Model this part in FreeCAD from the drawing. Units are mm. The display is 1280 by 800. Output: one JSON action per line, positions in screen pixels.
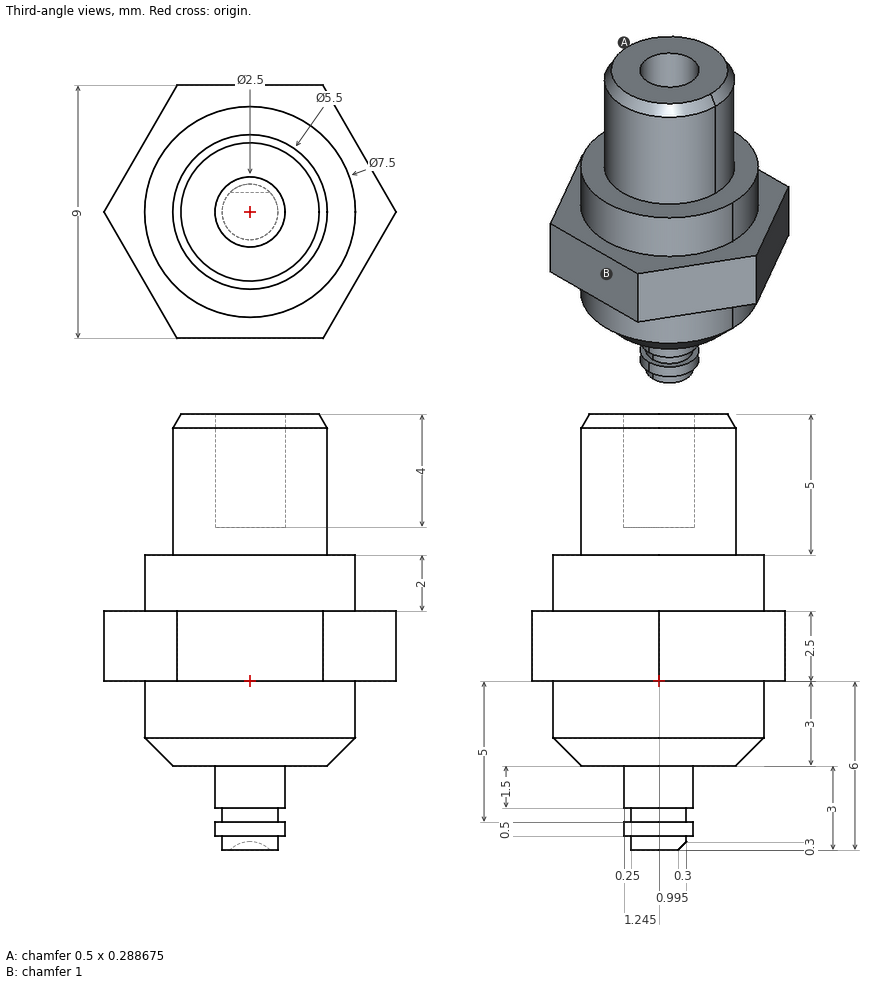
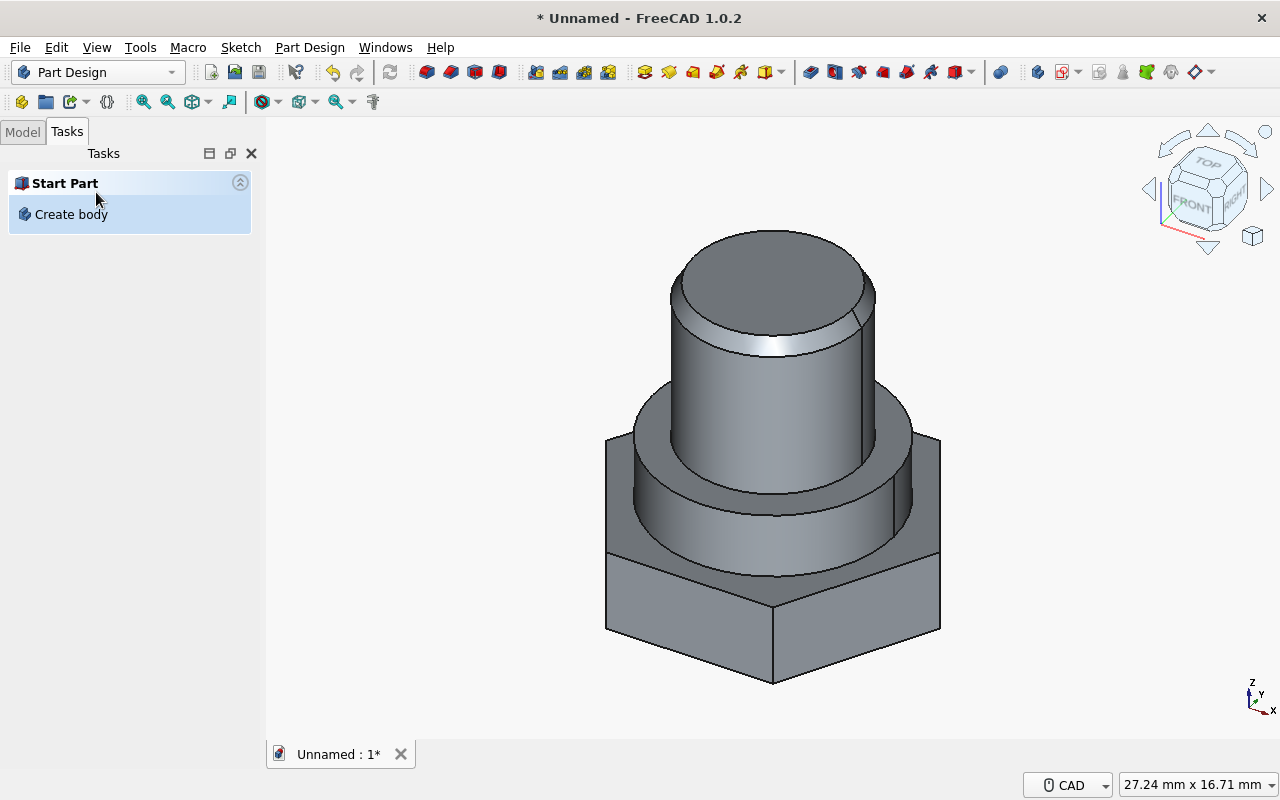
{"action": "left_click", "coordinate": [773, 282]}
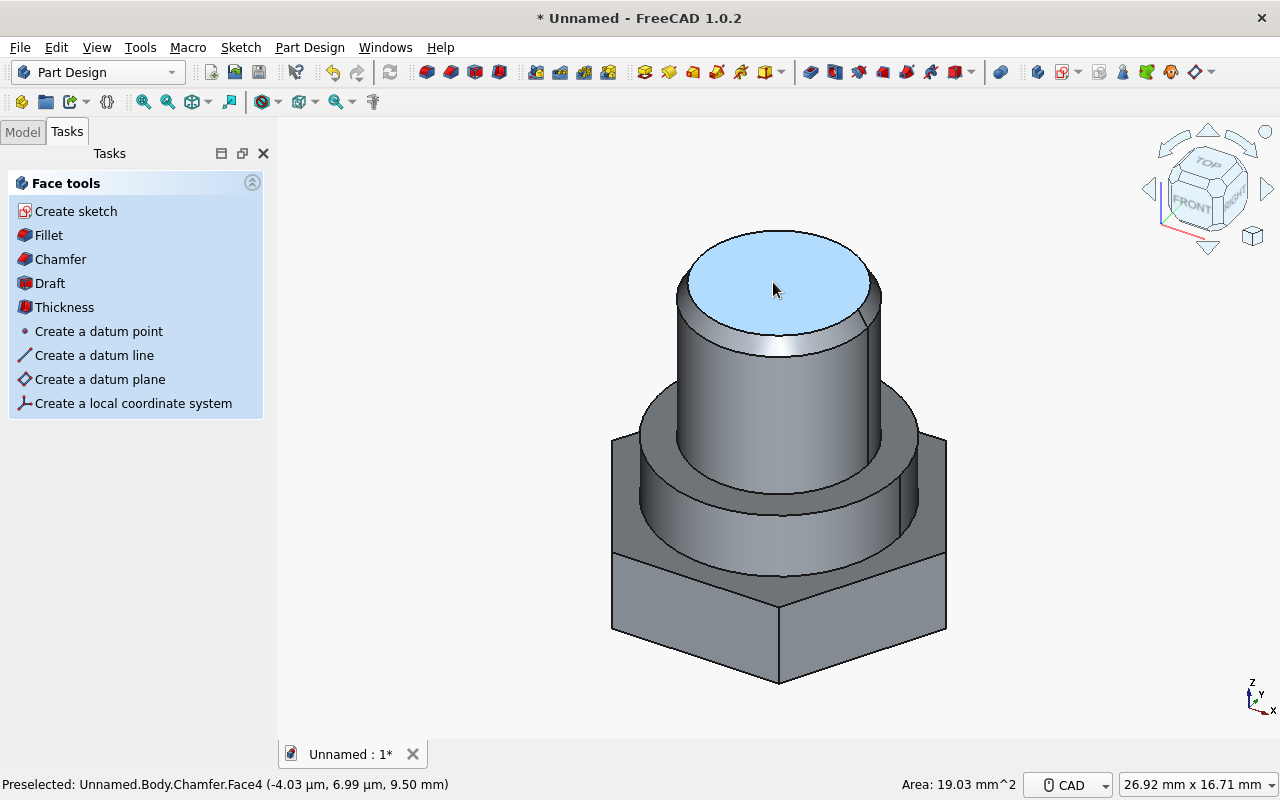
{"action": "left_click", "coordinate": [1062, 72]}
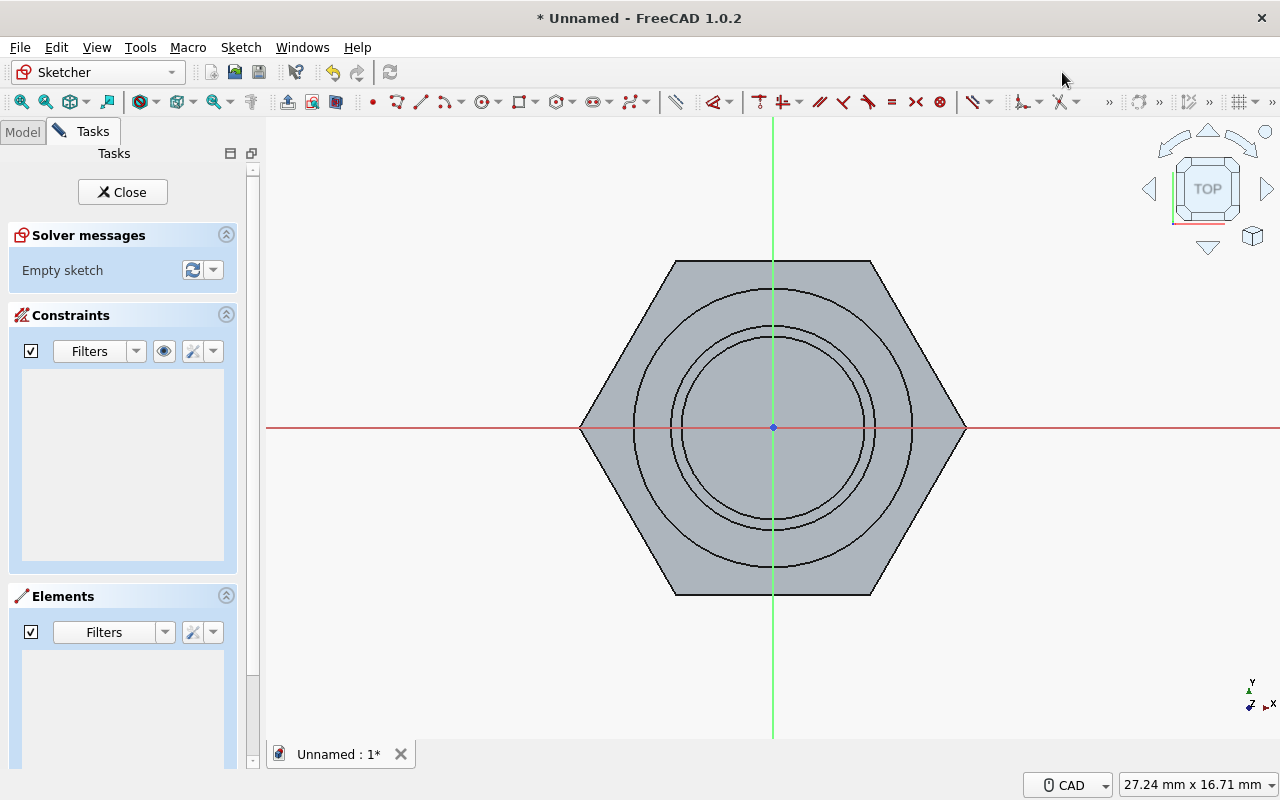
{"action": "scroll", "coordinate": [795, 428], "scroll_direction": "up", "scroll_amount": 7}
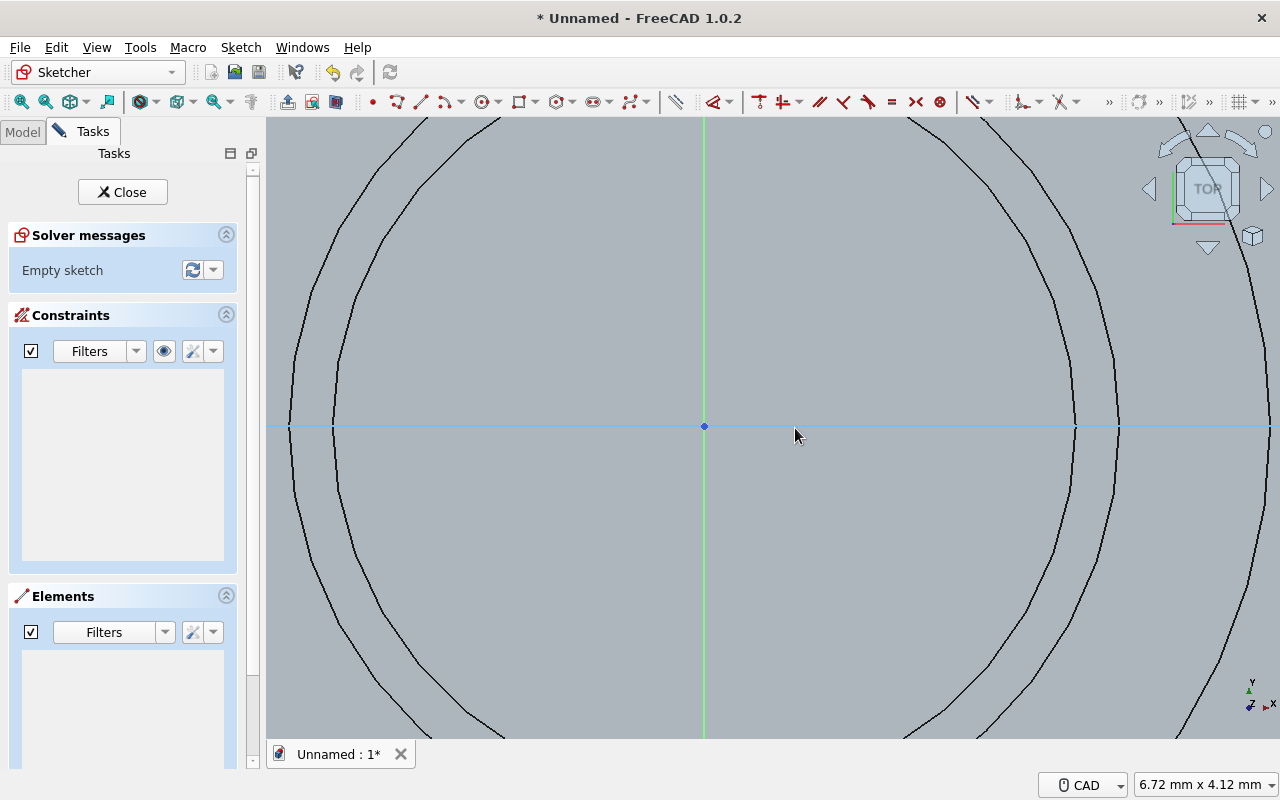
{"action": "key", "text": "g c"}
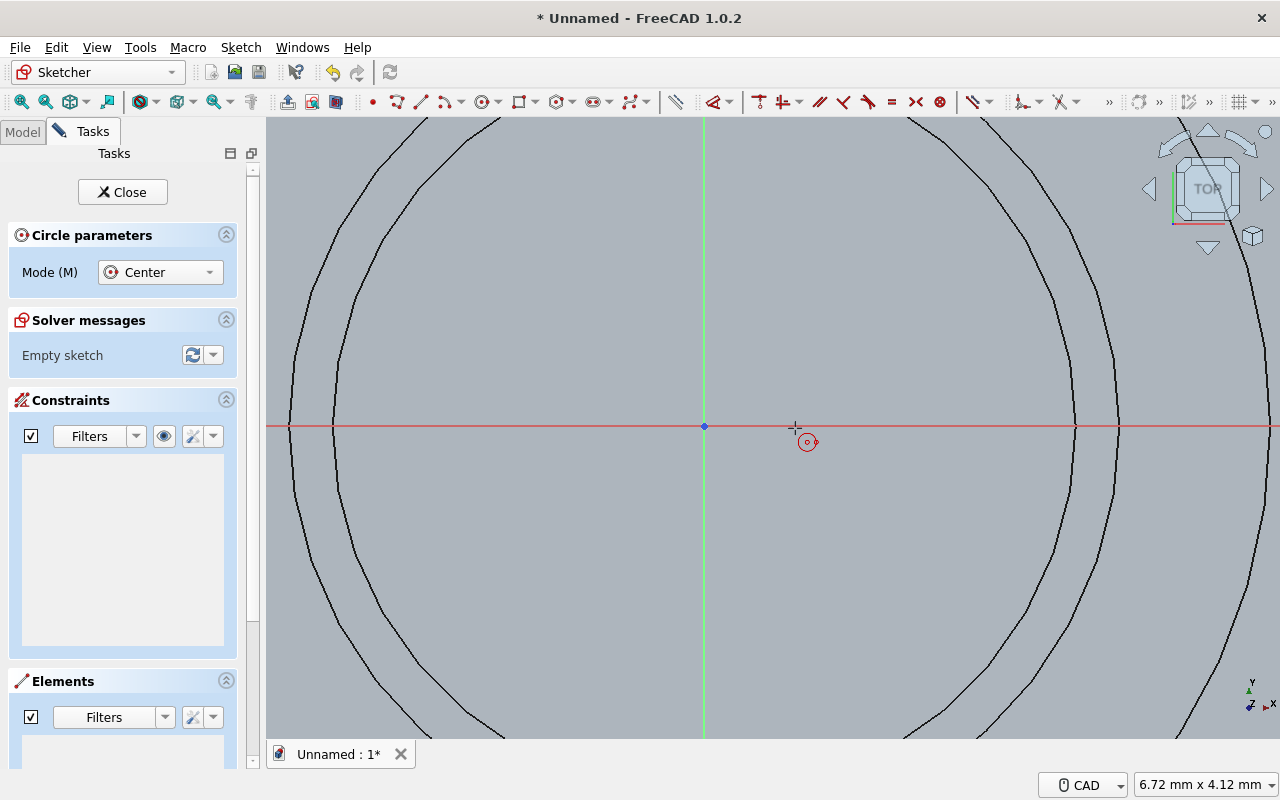
{"action": "left_click", "coordinate": [704, 426]}
{"action": "left_click", "coordinate": [838, 293]}
{"action": "key", "text": "Escape"}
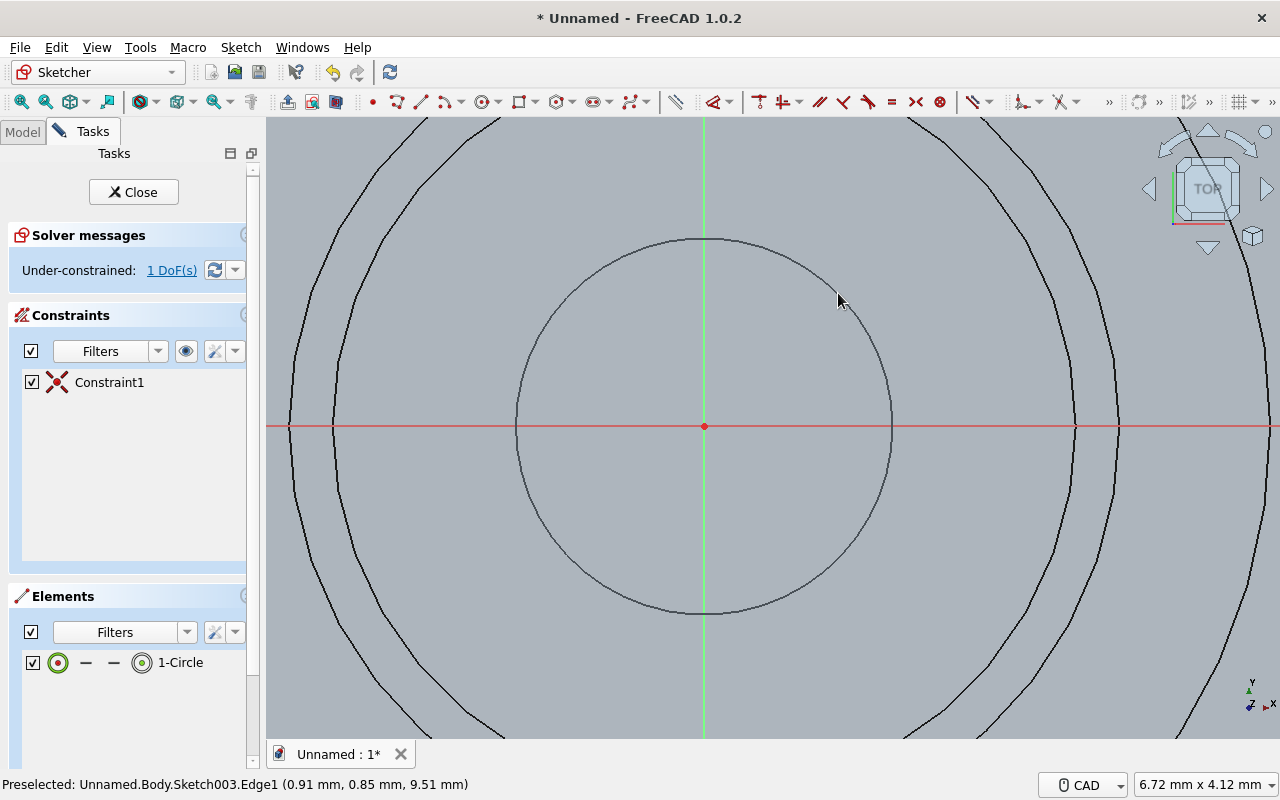
{"action": "left_click", "coordinate": [837, 293]}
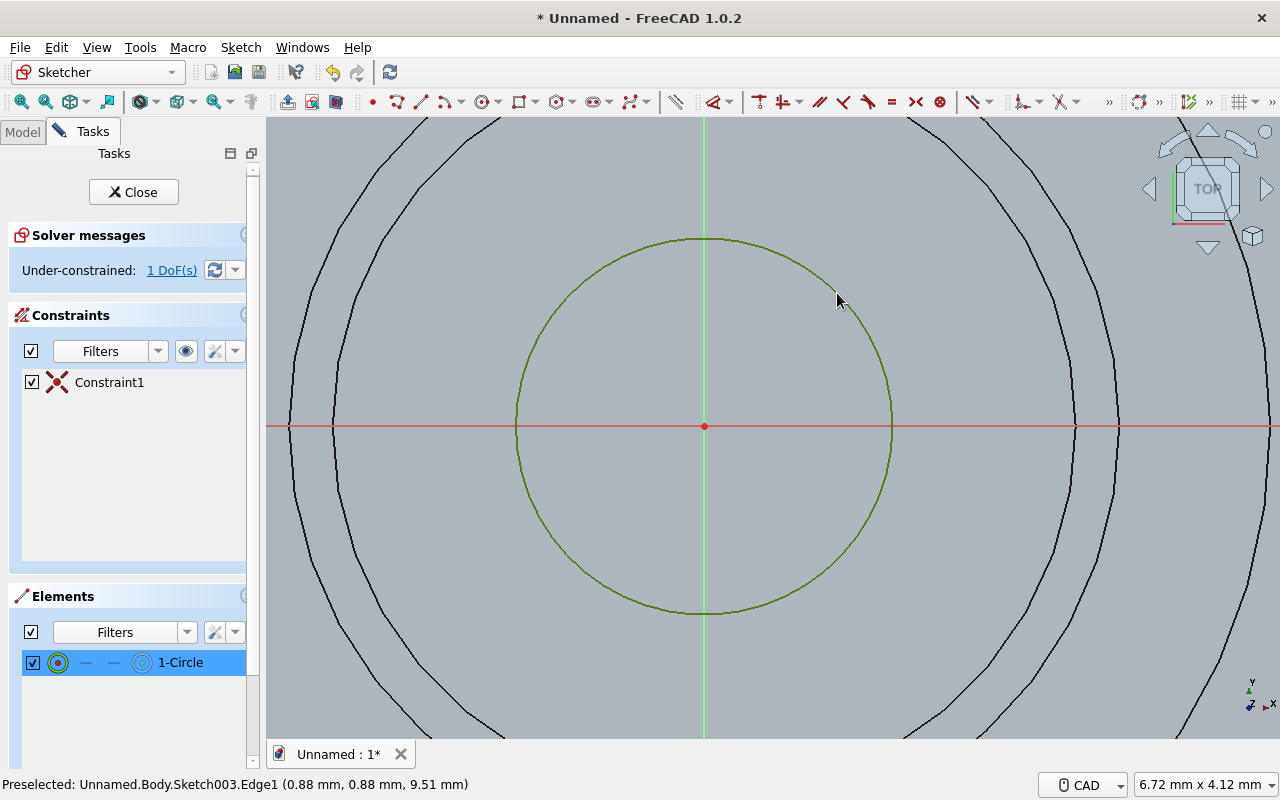
{"action": "key", "text": "k o"}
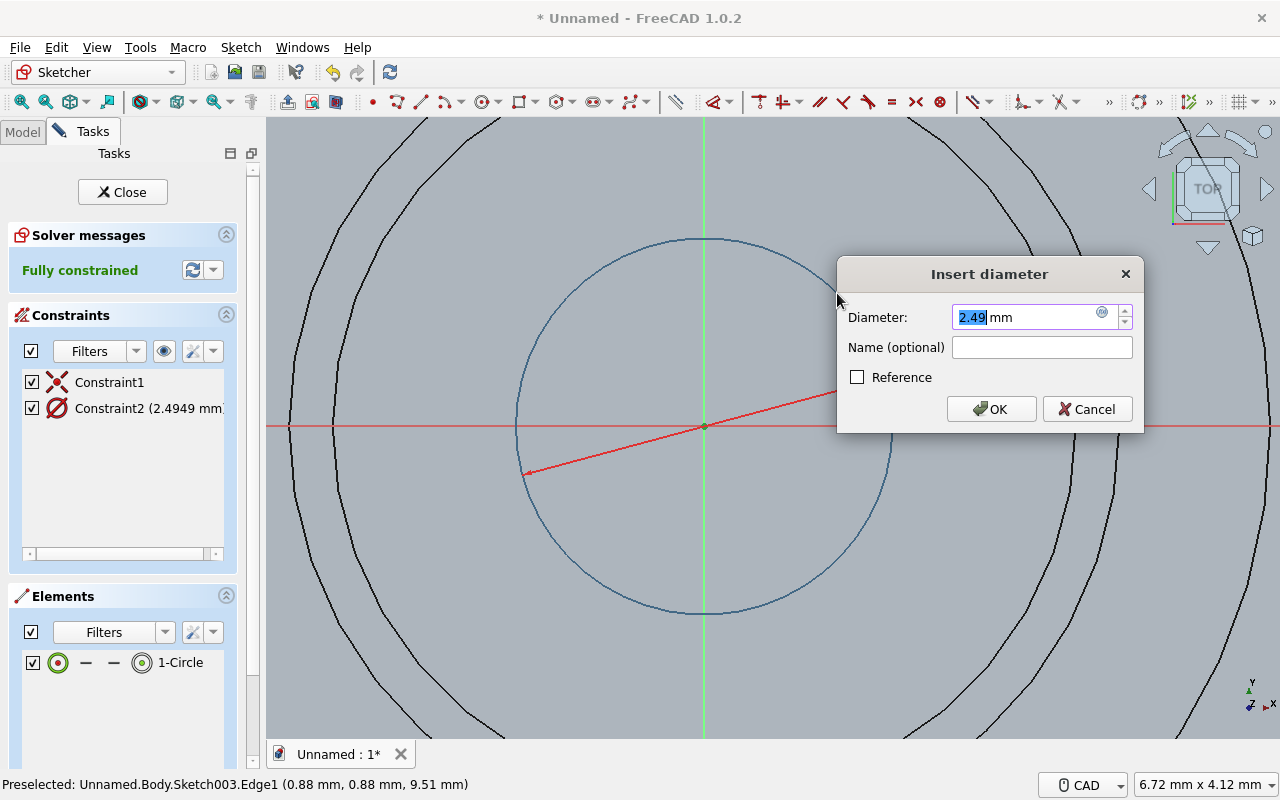
{"action": "type", "text": "2.5"}
{"action": "key", "text": "Return"}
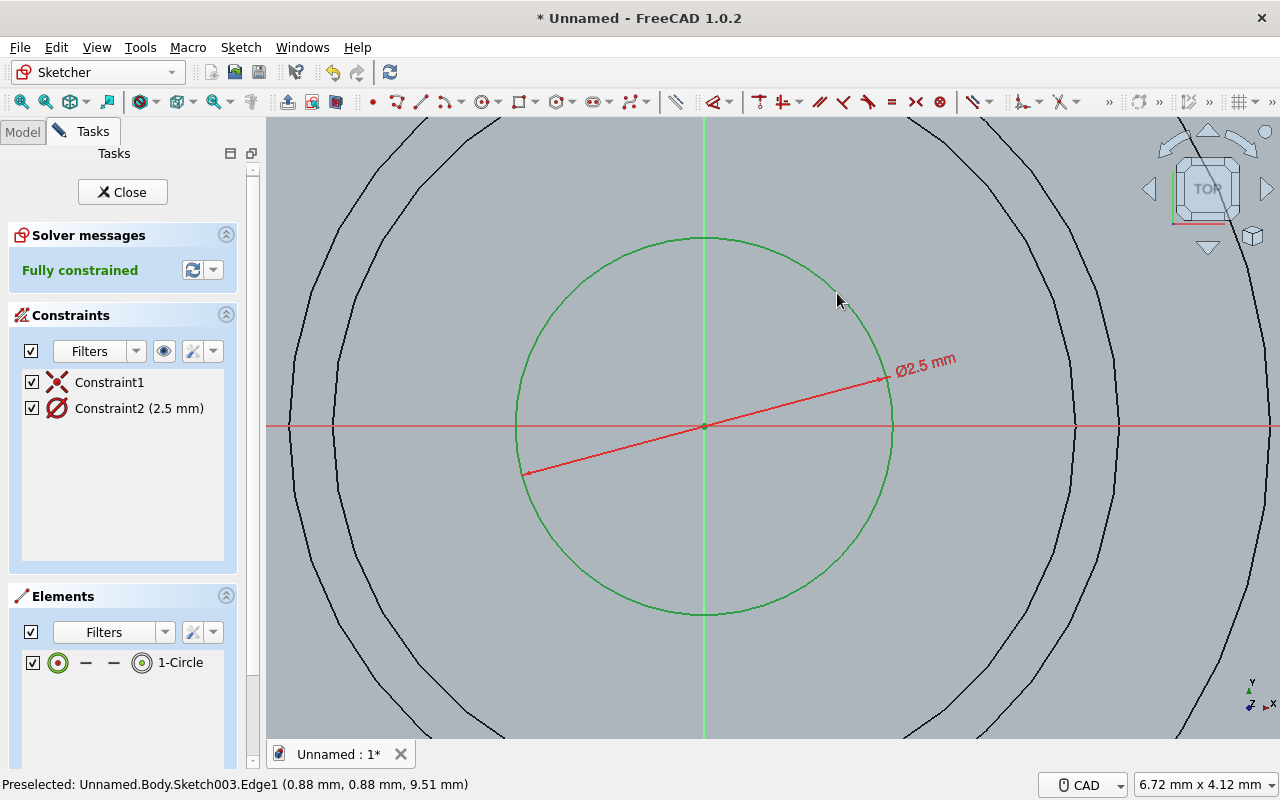
{"action": "left_click", "coordinate": [123, 192]}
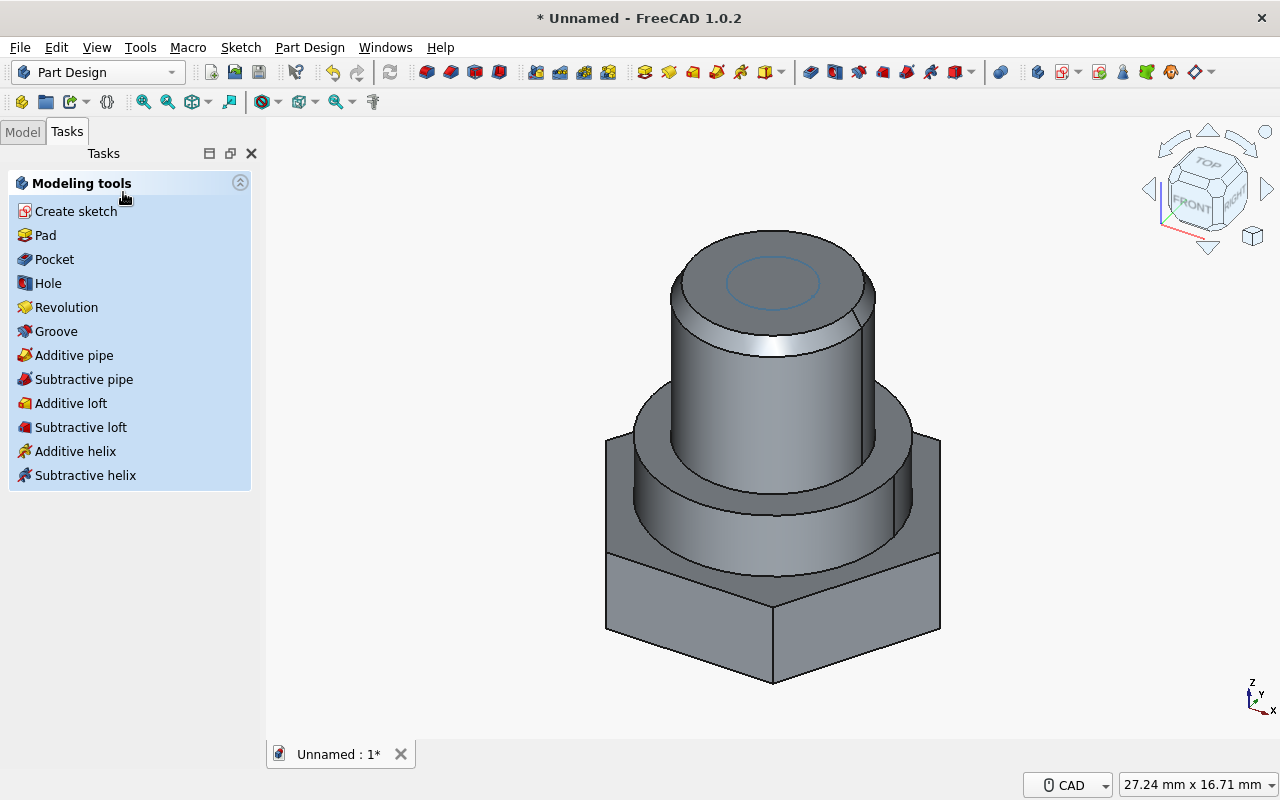
{"action": "left_click", "coordinate": [812, 72]}